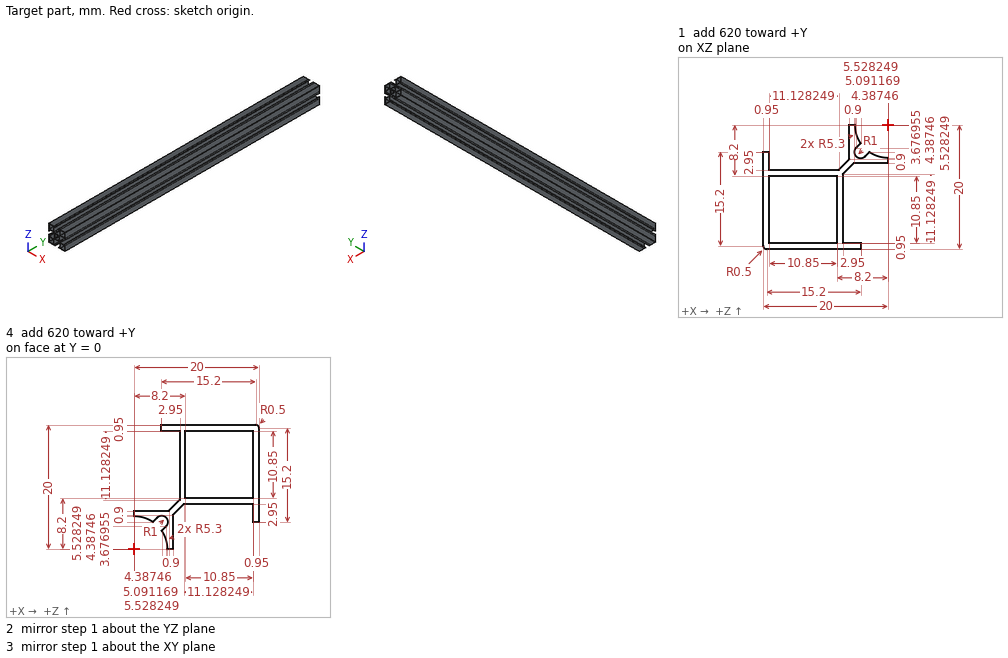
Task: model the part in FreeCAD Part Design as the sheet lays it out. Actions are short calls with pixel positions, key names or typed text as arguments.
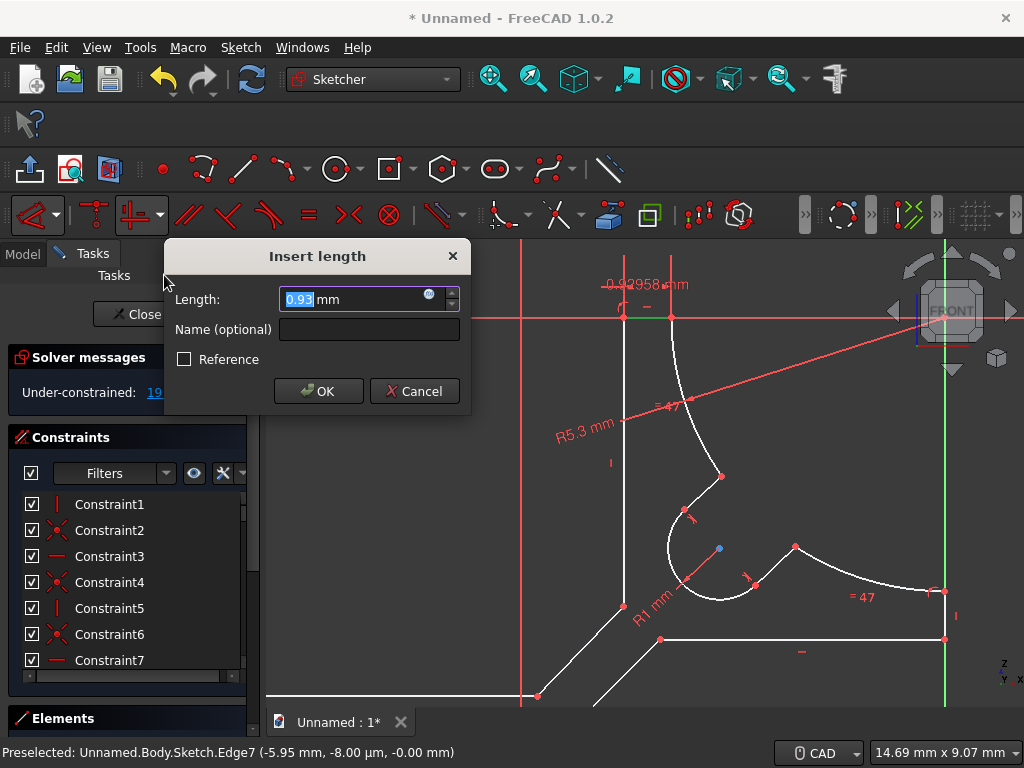
text(0.9)
key(Return)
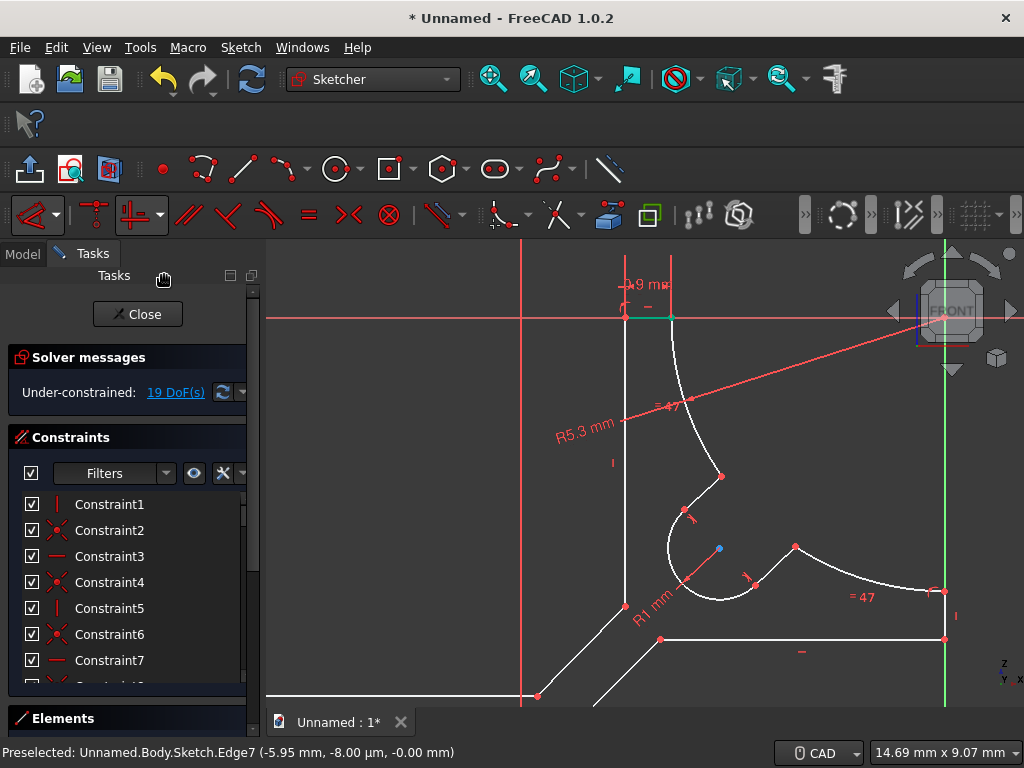
scroll(640, 318, down, 6)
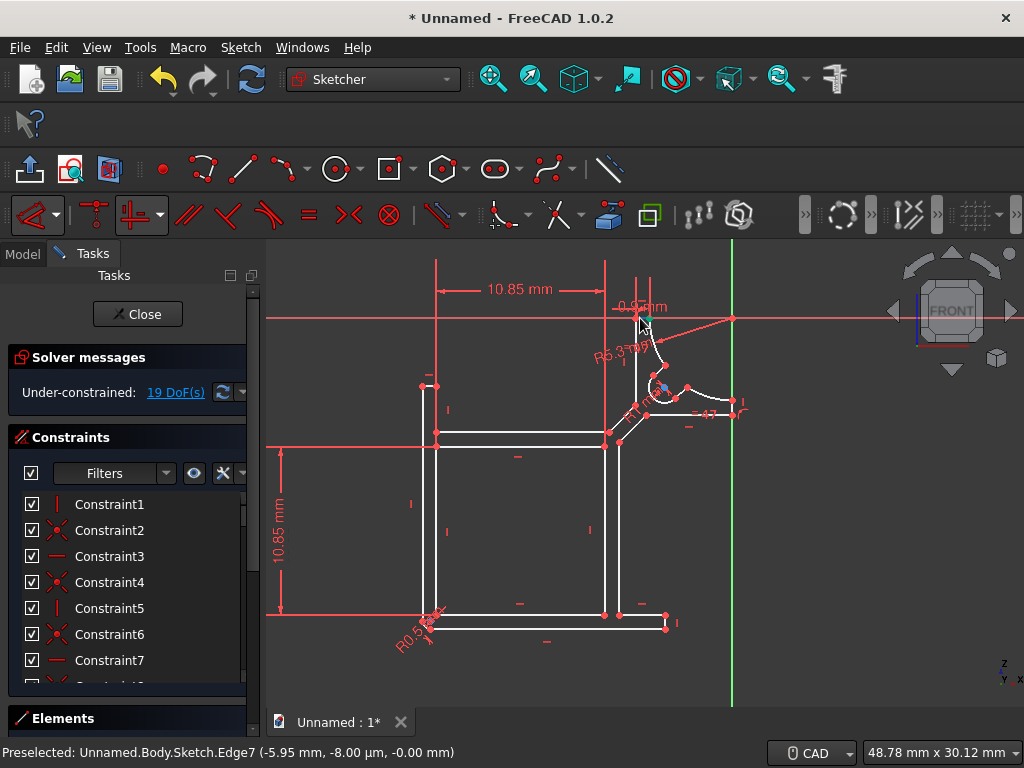
scroll(732, 405, up, 6)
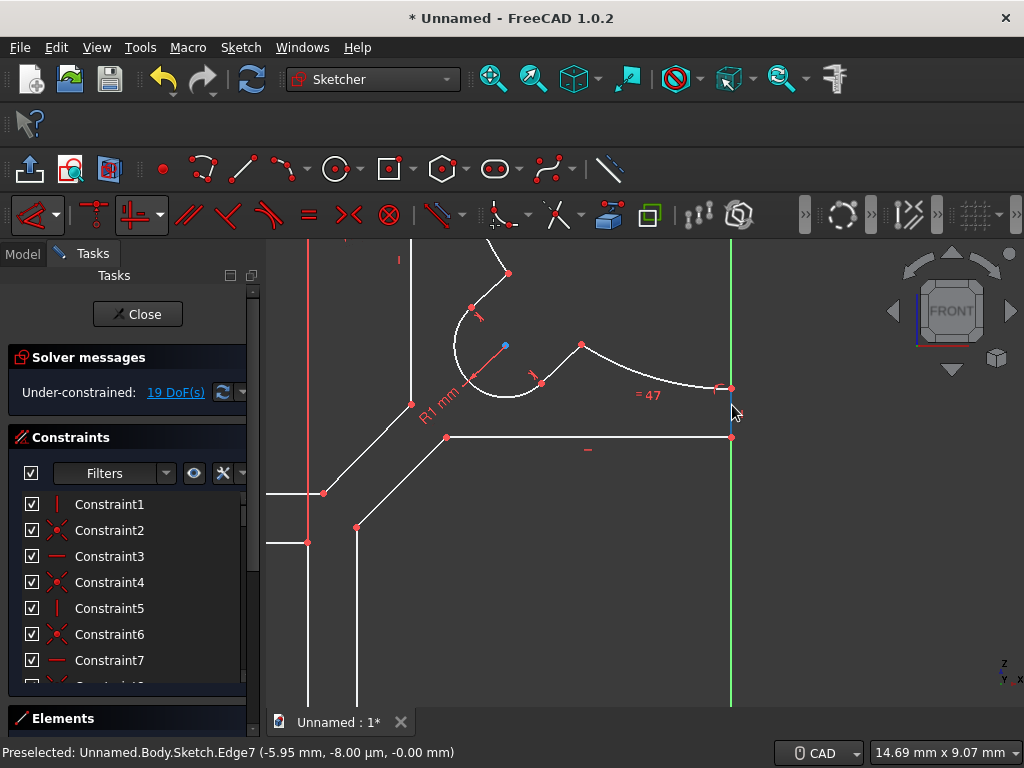
click(731, 403)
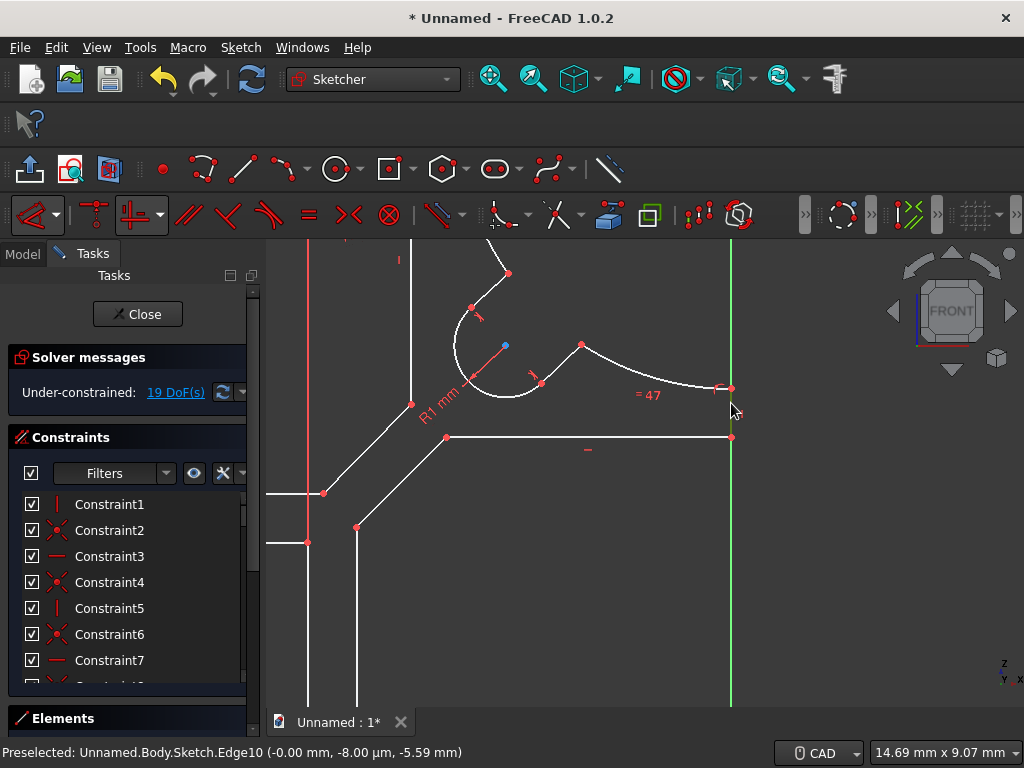
click(58, 216)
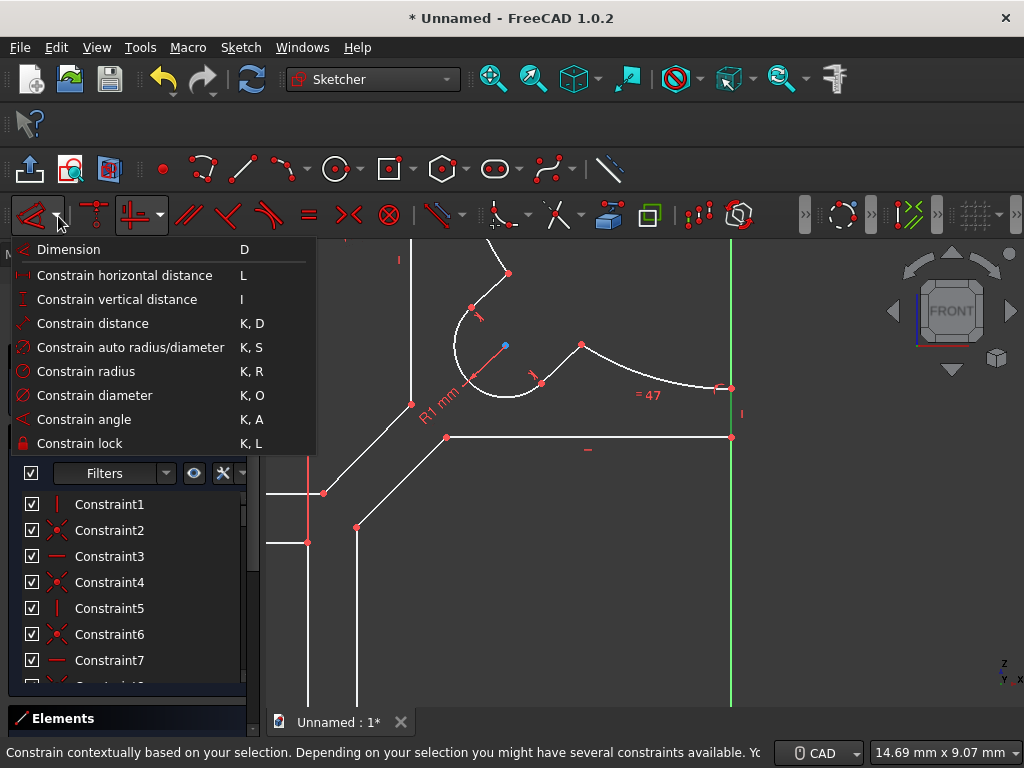
click(164, 299)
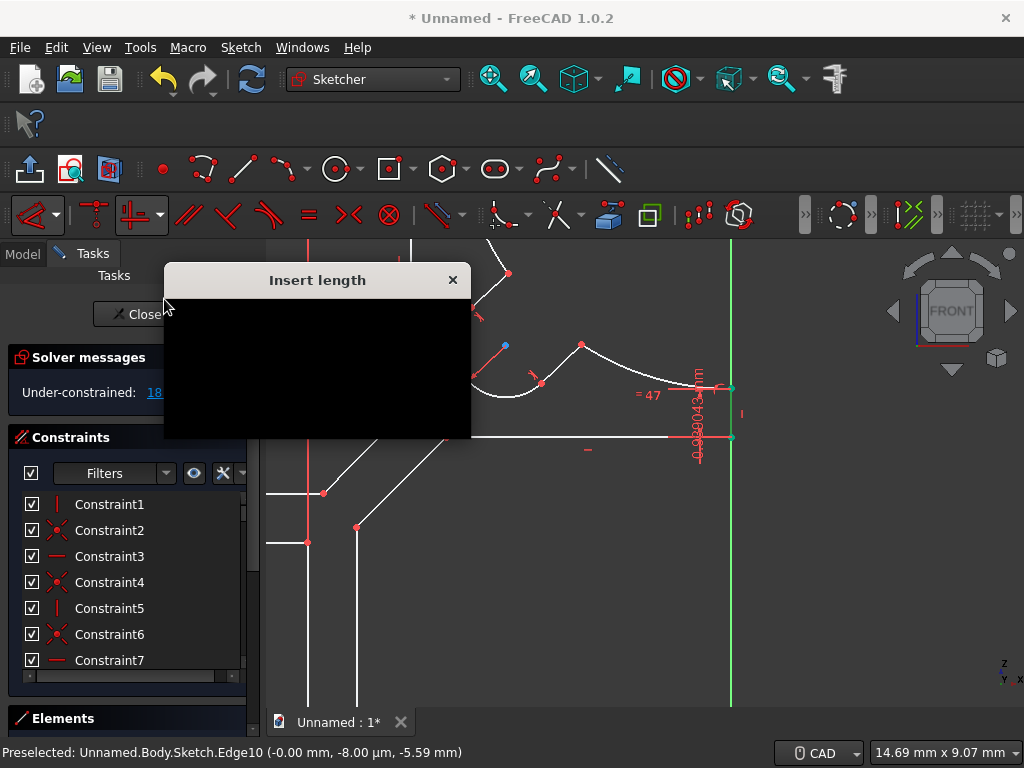
text(0.9)
key(Return)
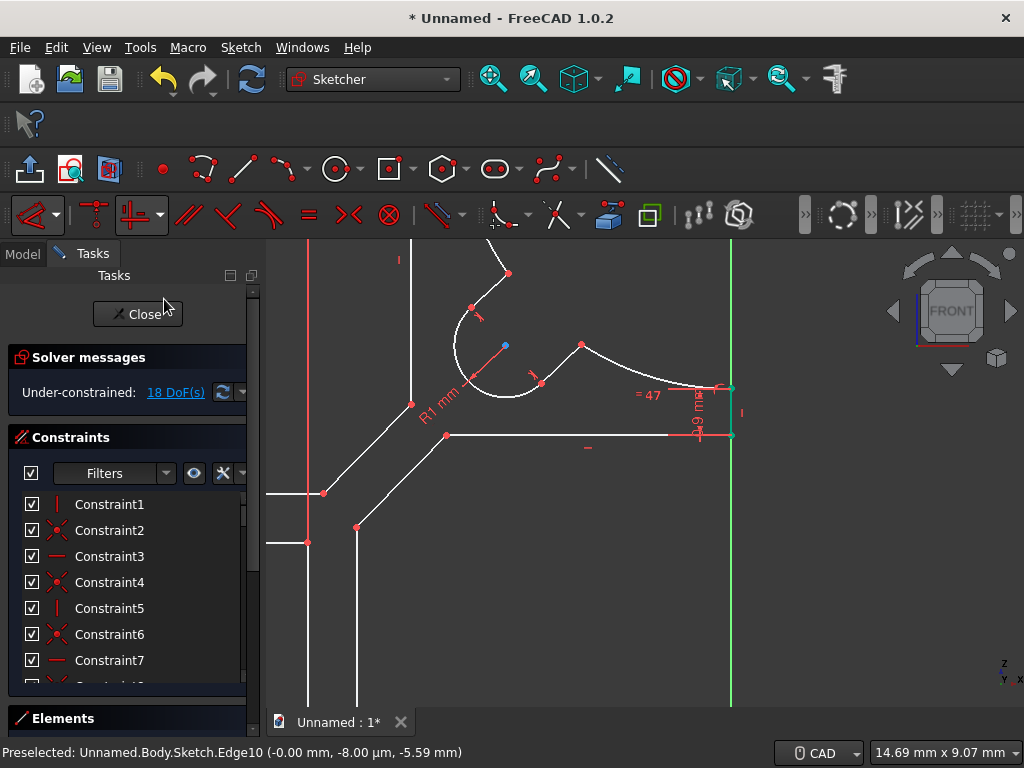
scroll(732, 405, down, 6)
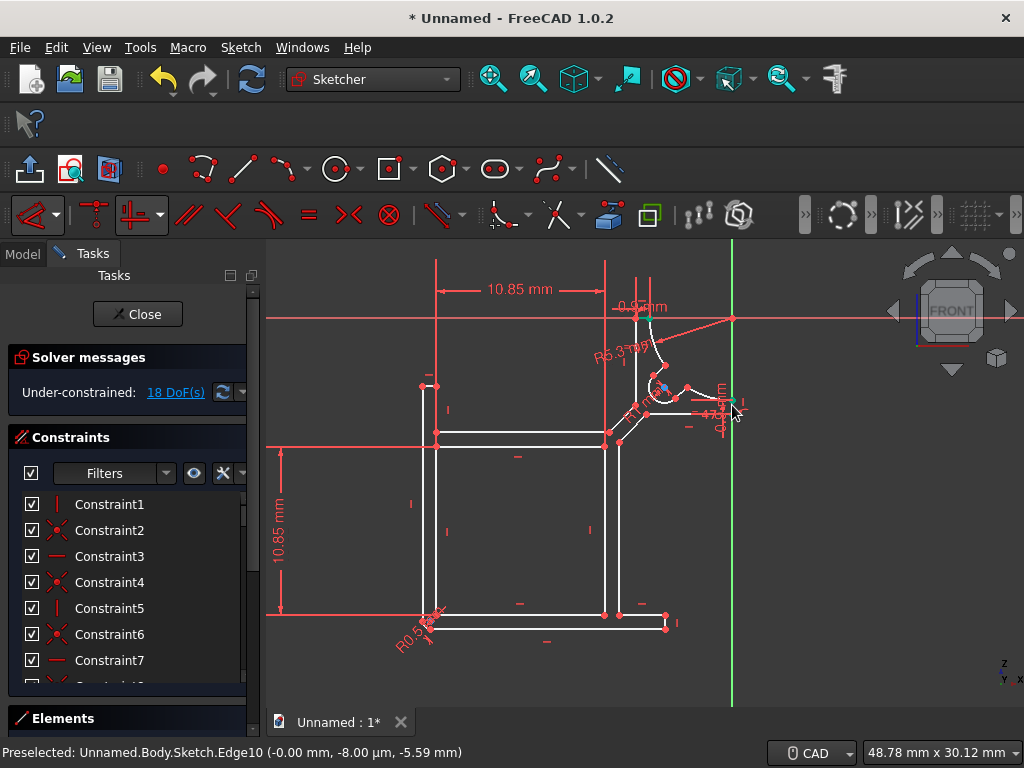
scroll(423, 622, up, 3)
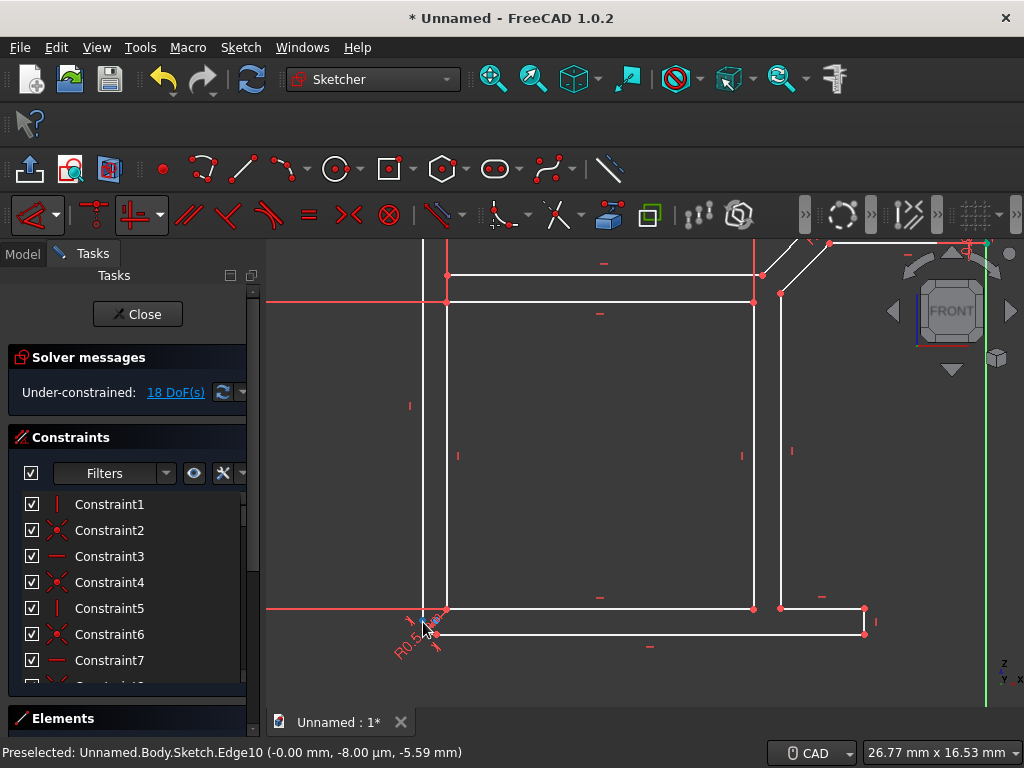
click(423, 621)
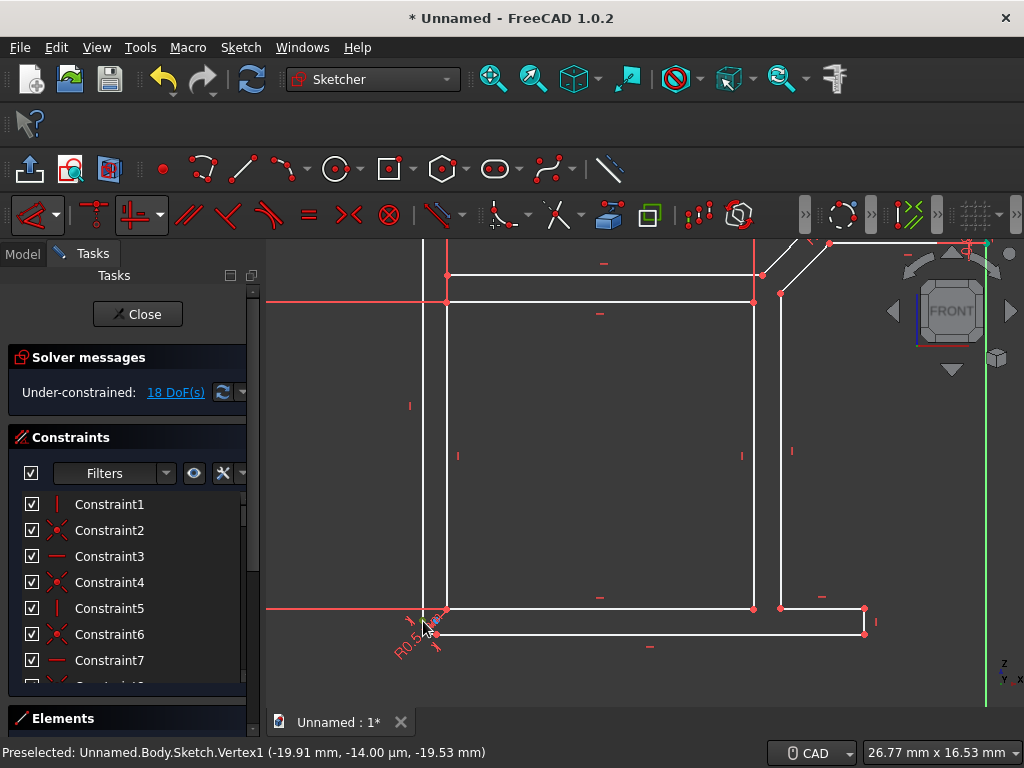
key(l)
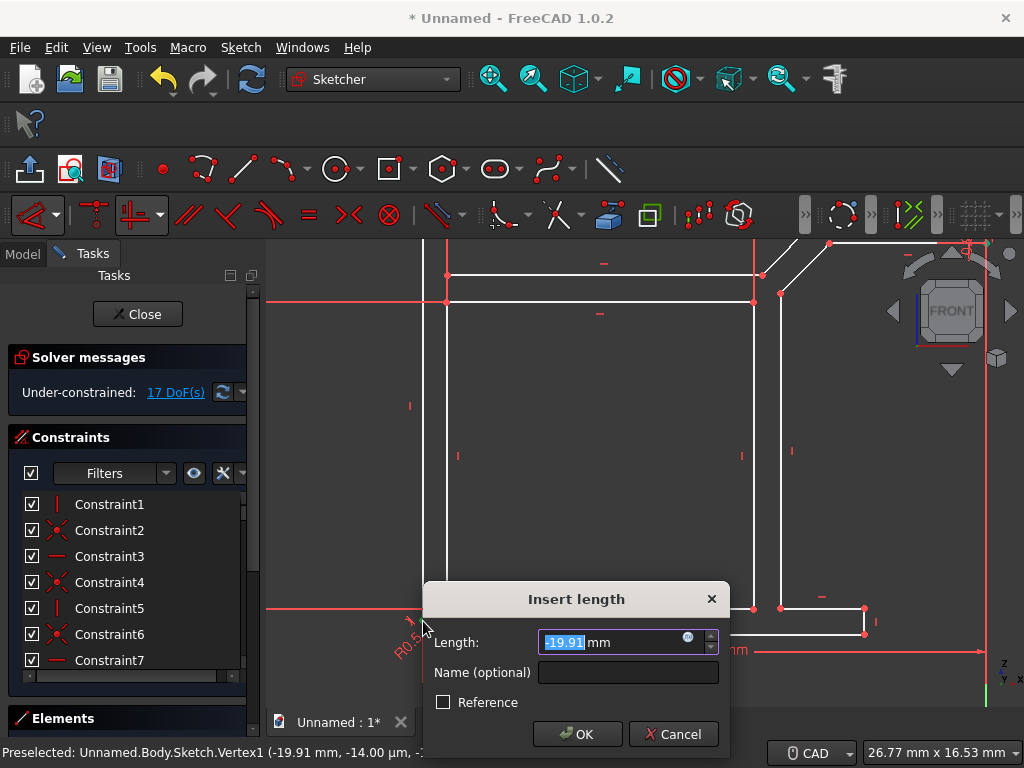
text(-20)
key(Return)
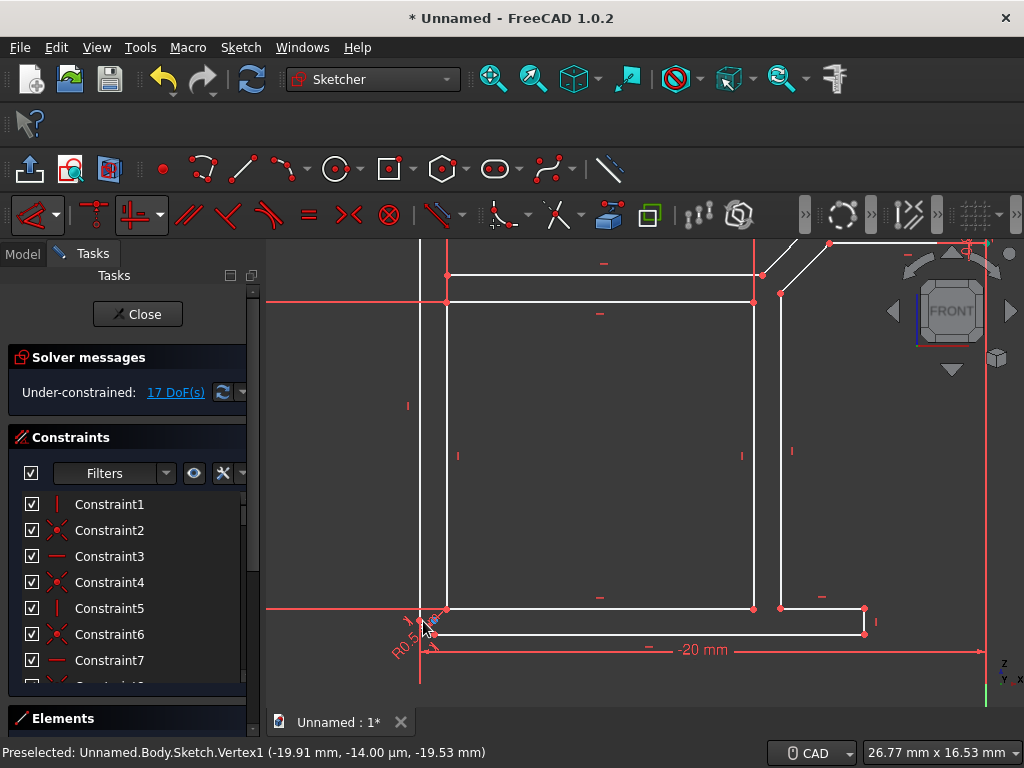
scroll(423, 622, down, 3)